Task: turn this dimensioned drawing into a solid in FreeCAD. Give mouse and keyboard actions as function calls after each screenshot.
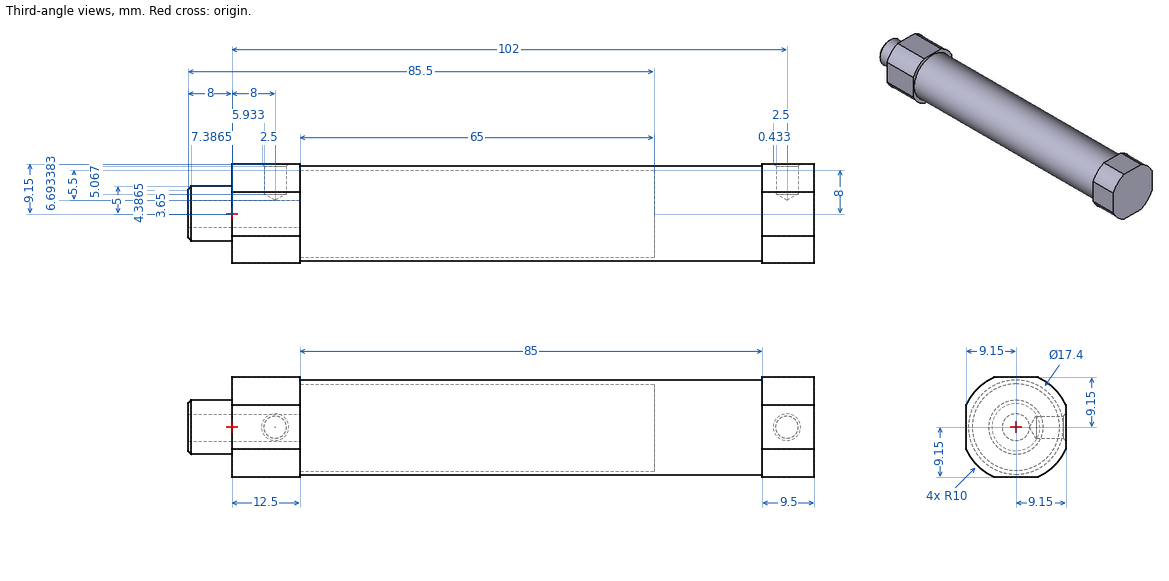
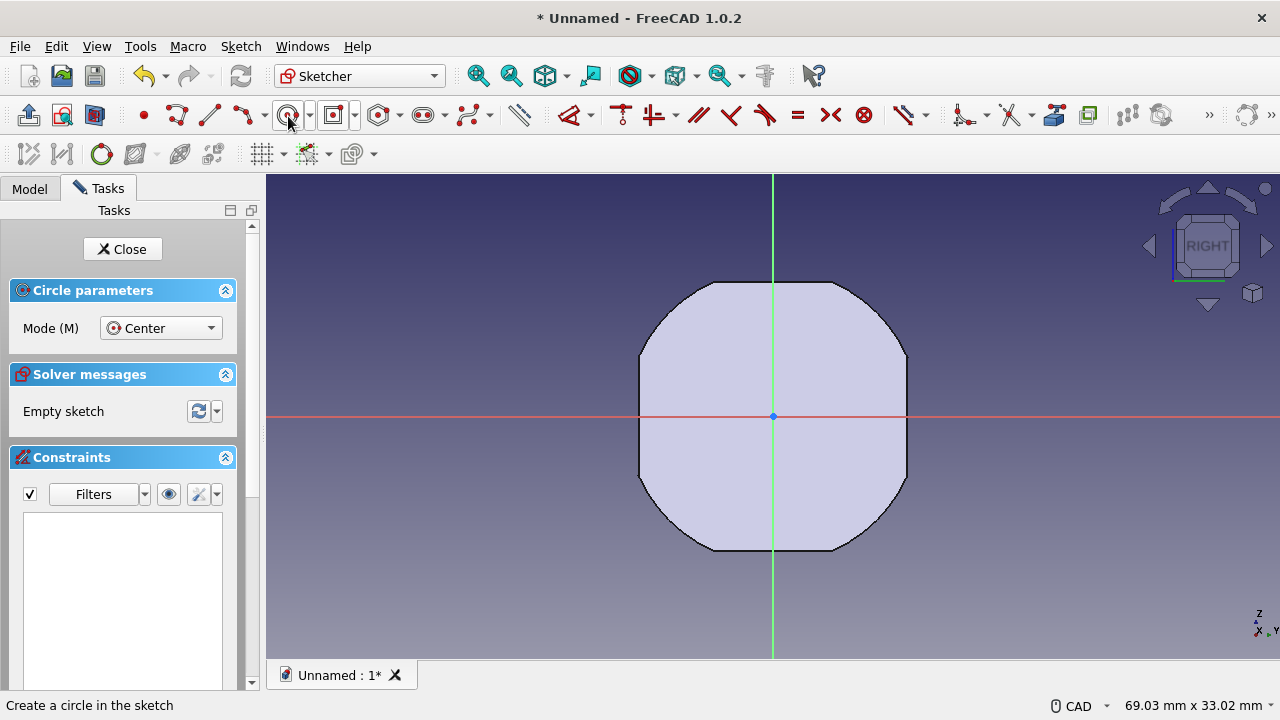
click(773, 416)
move(863, 326)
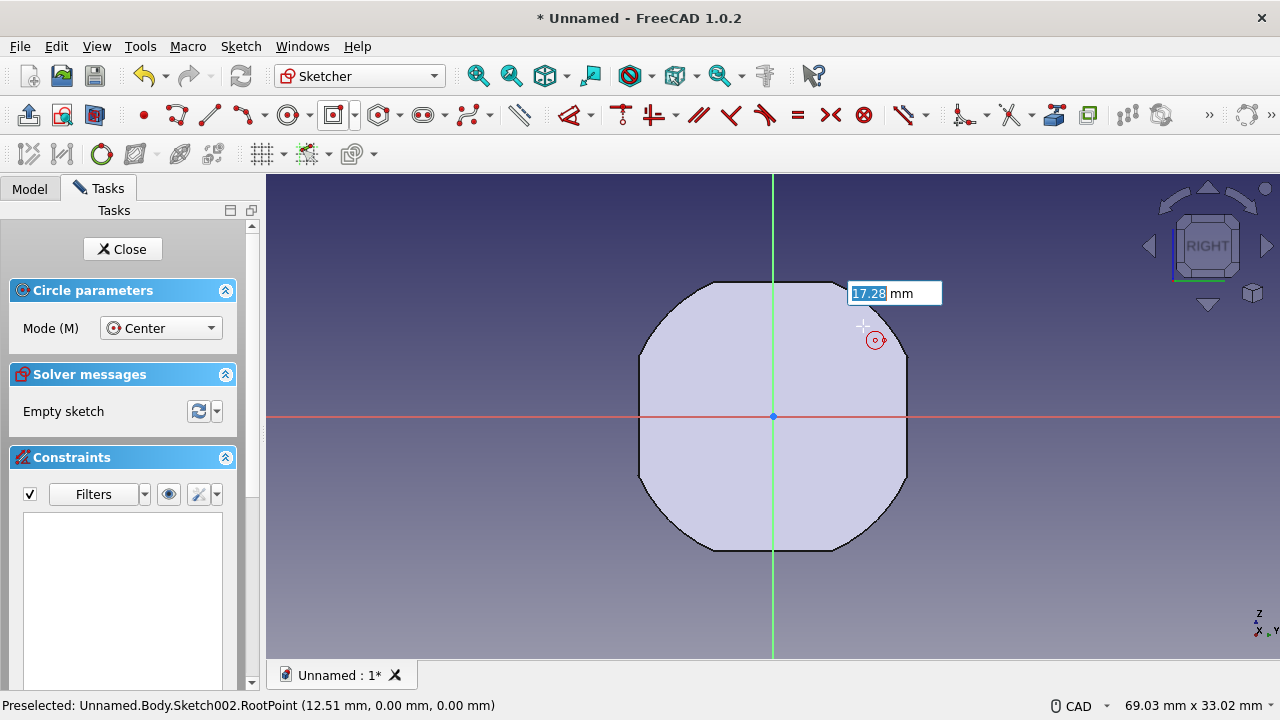
text(17.4)
key(Return)
key(Escape)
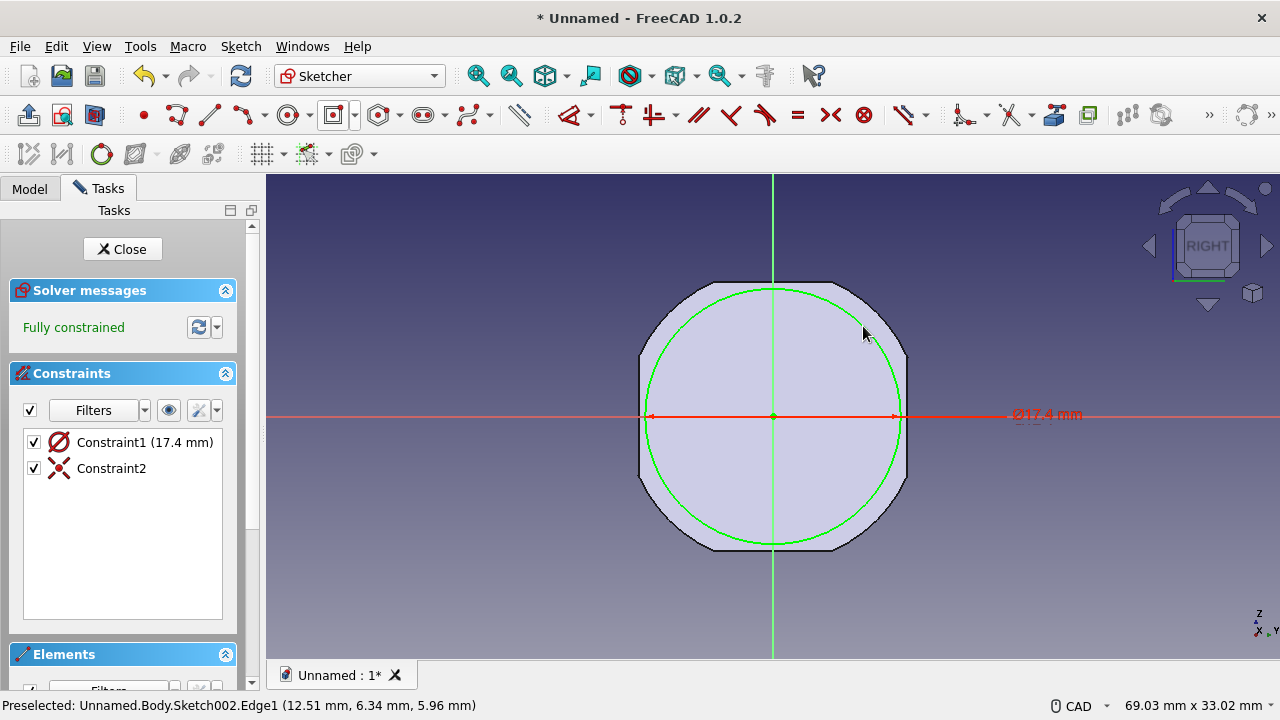
click(123, 249)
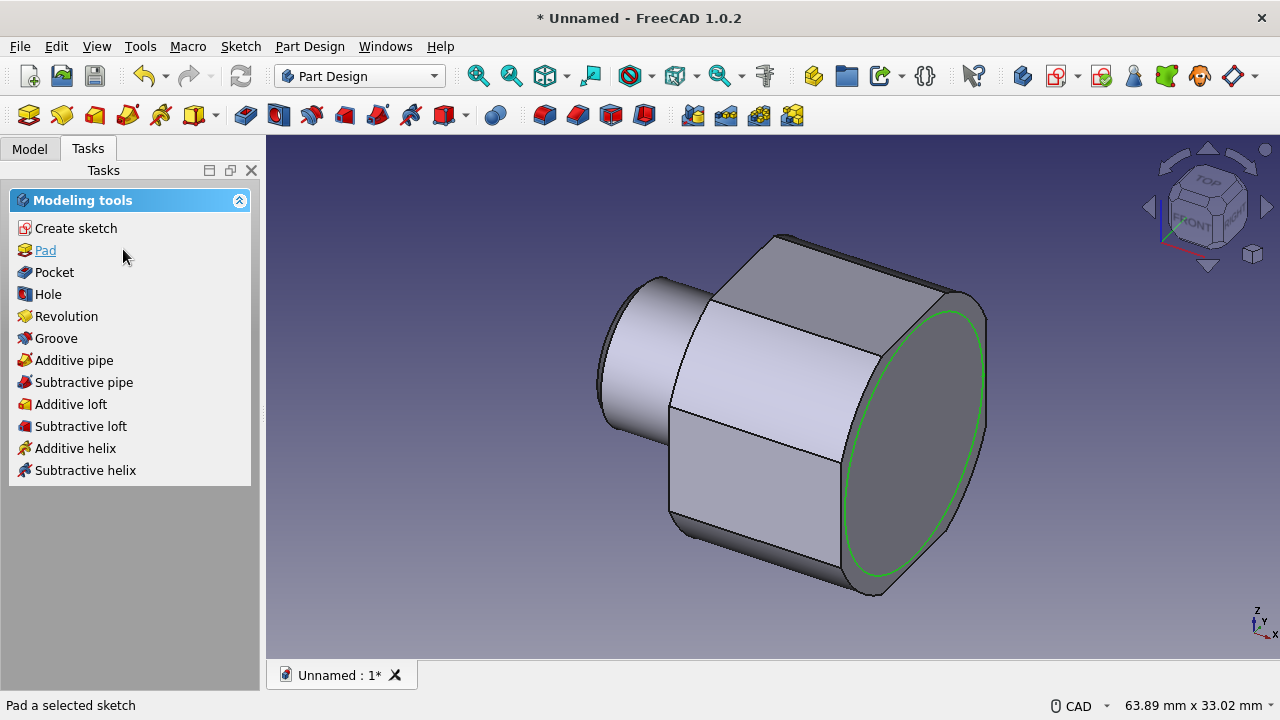
click(29, 116)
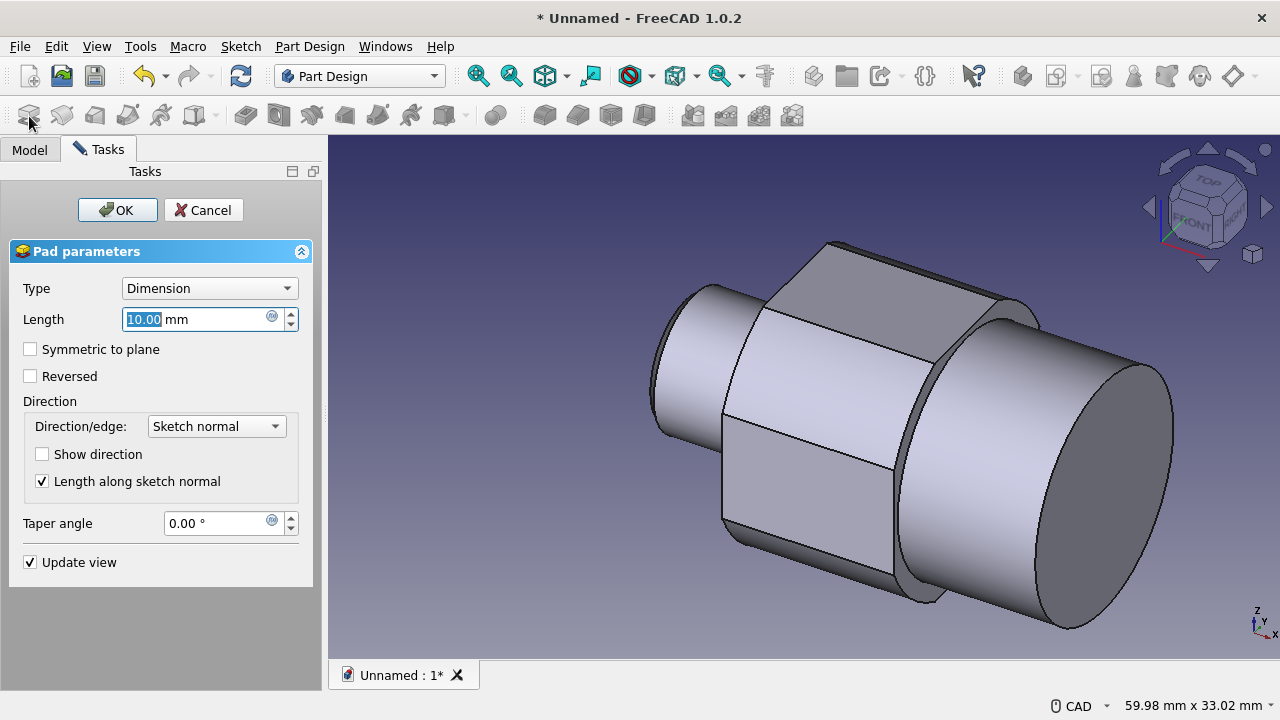
text(85)
key(Tab)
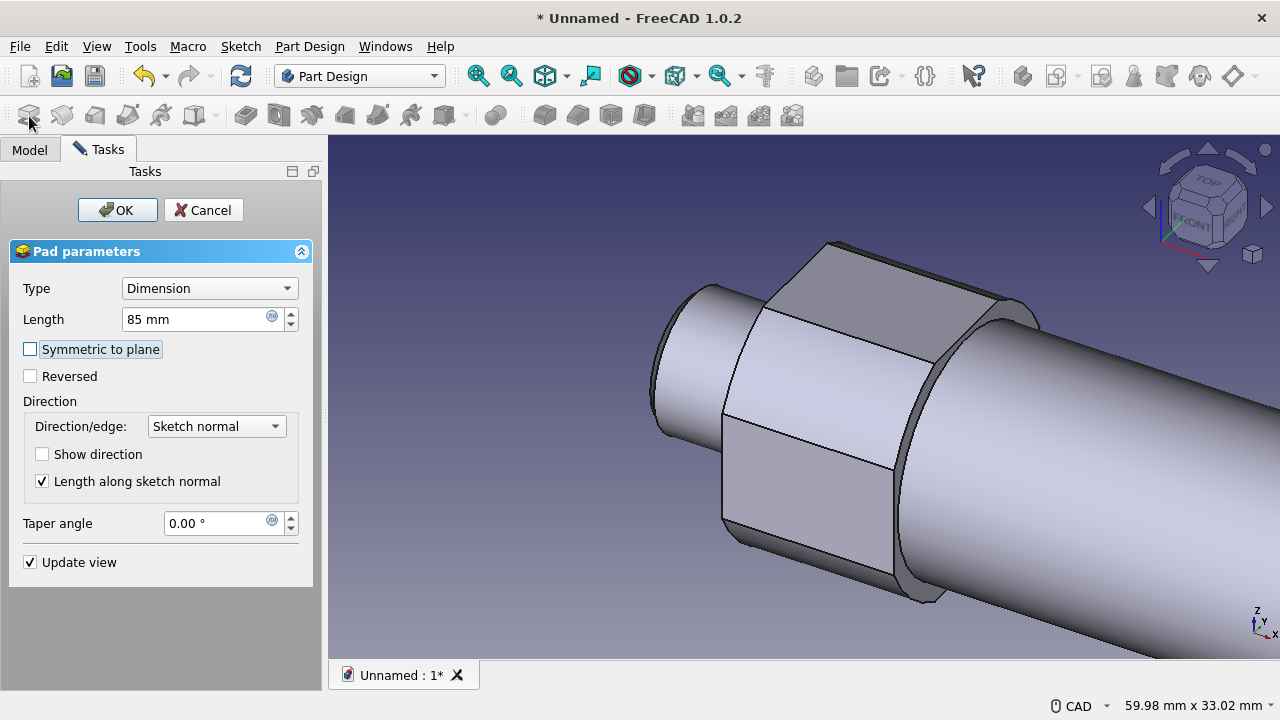
click(118, 210)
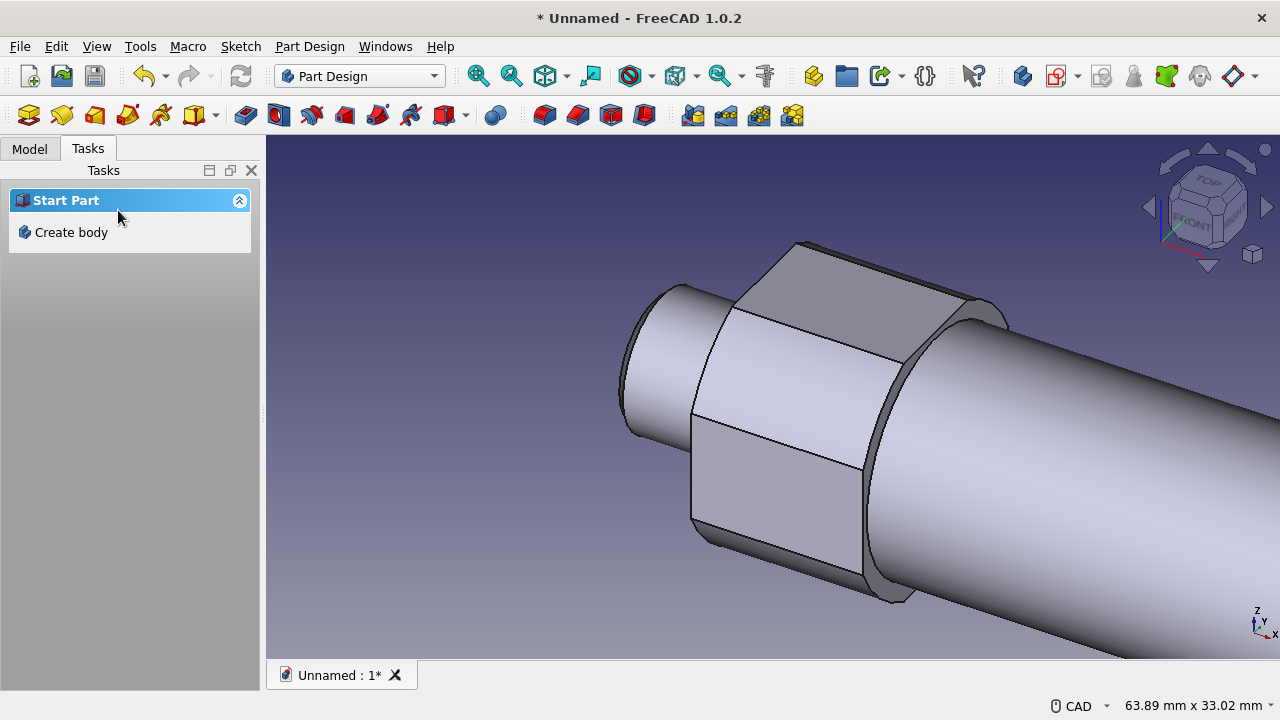
click(479, 76)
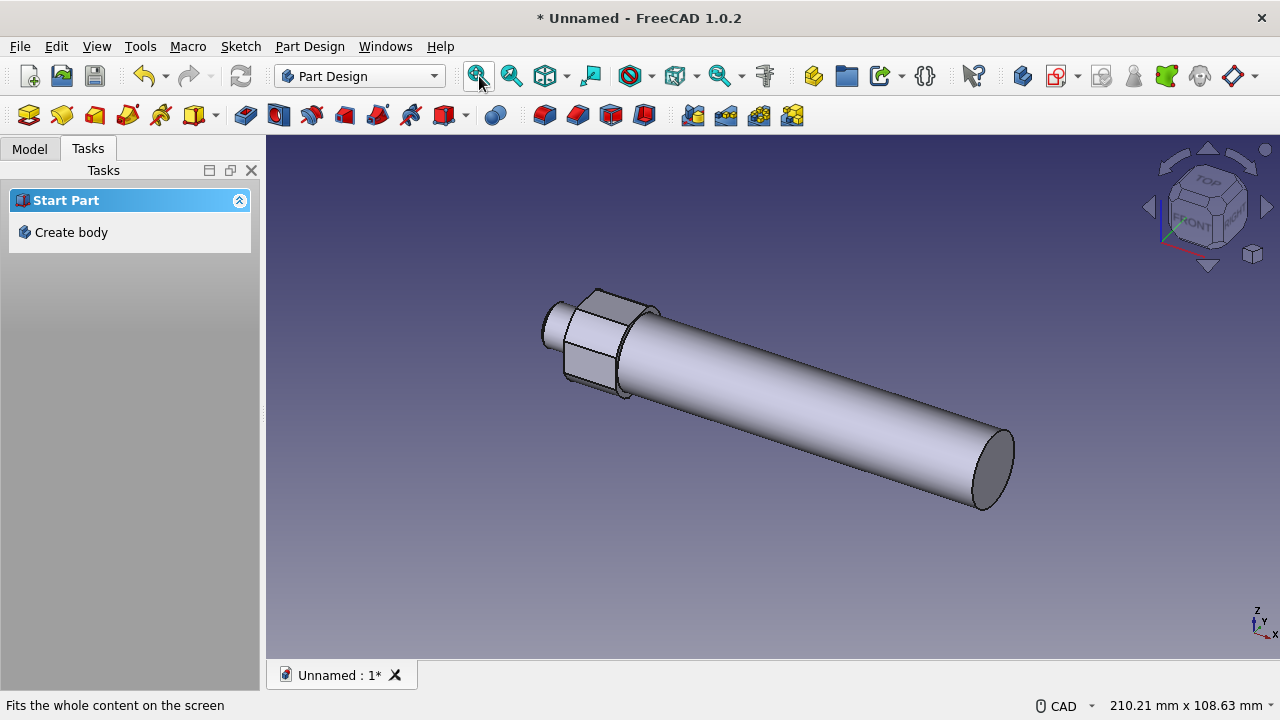
click(993, 469)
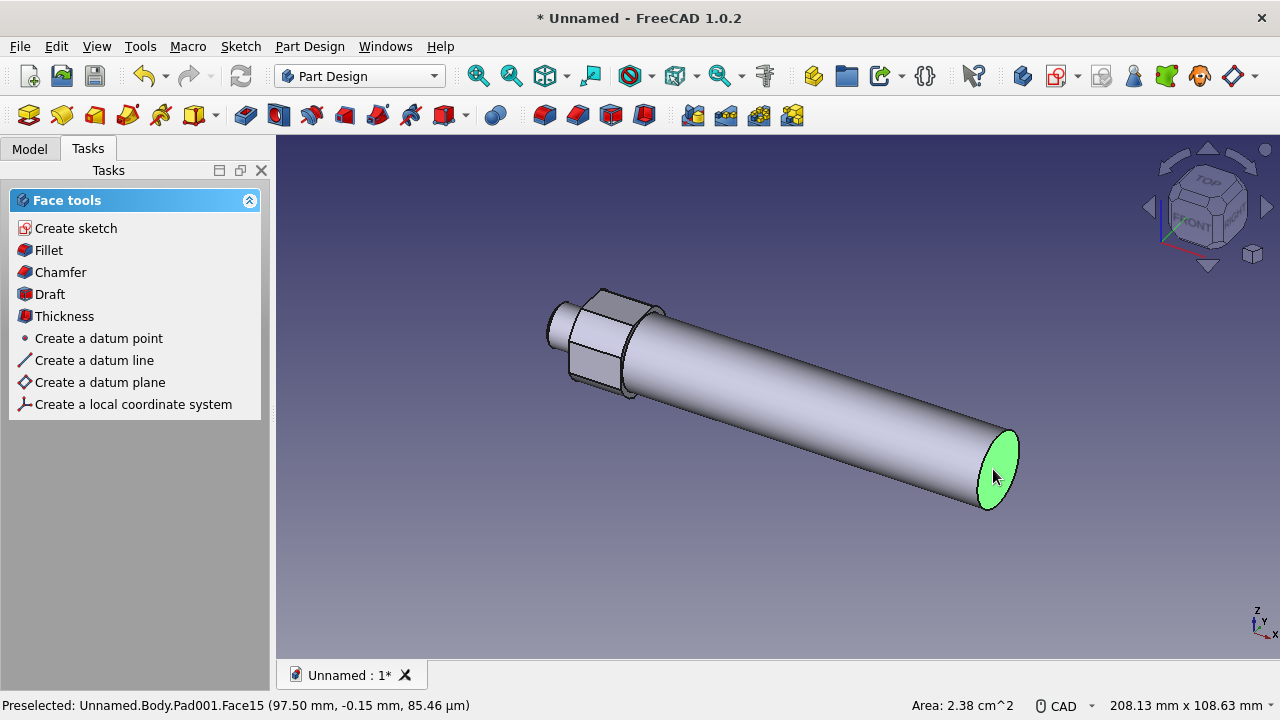
click(1056, 76)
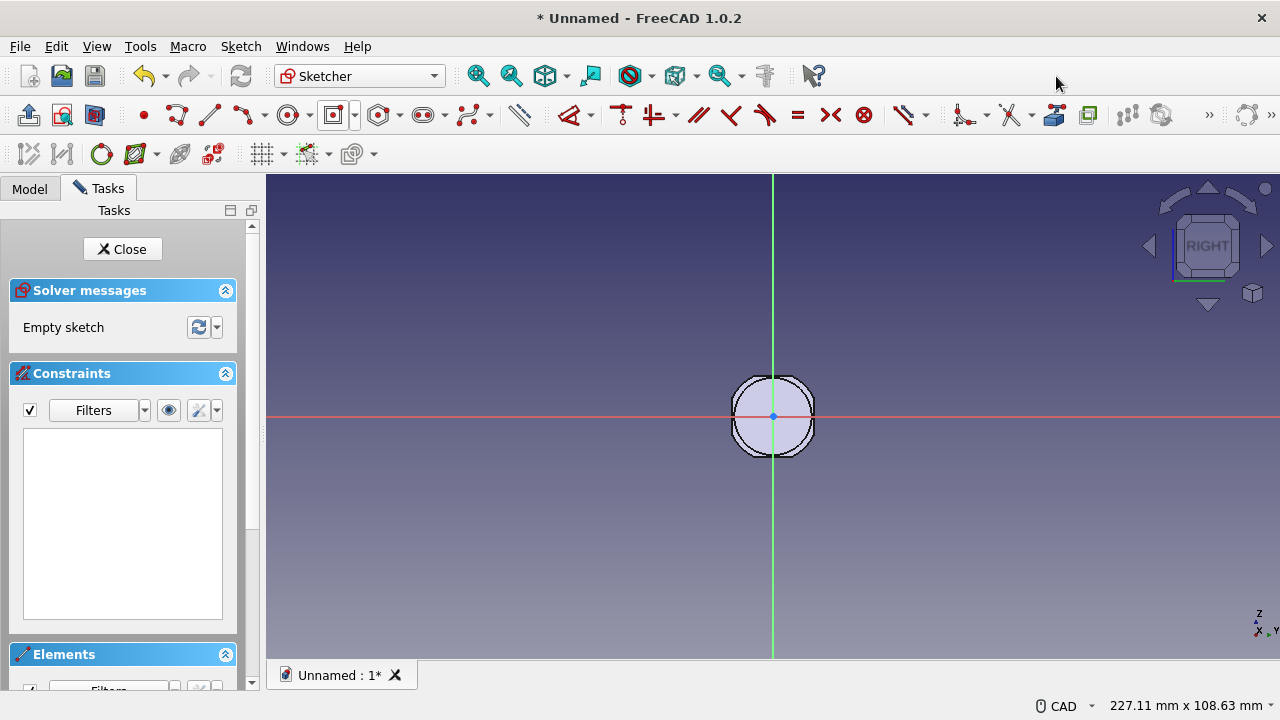
scroll(795, 416, up, 7)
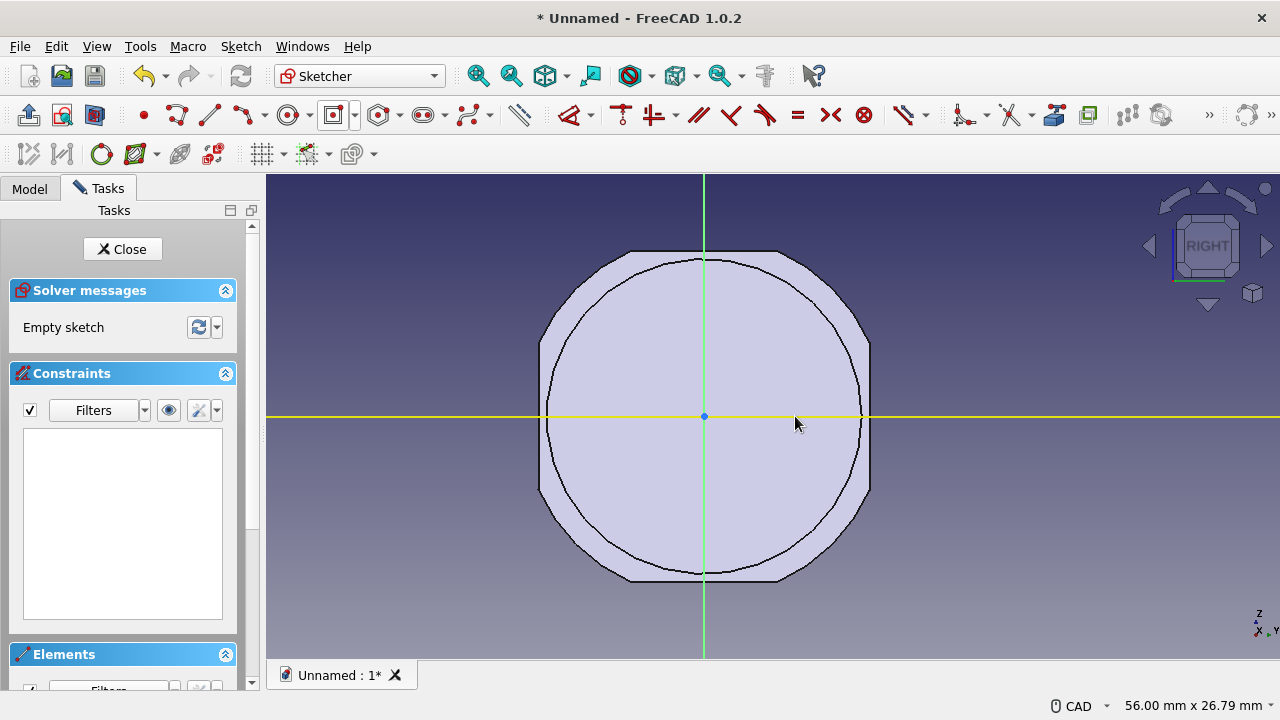
click(210, 116)